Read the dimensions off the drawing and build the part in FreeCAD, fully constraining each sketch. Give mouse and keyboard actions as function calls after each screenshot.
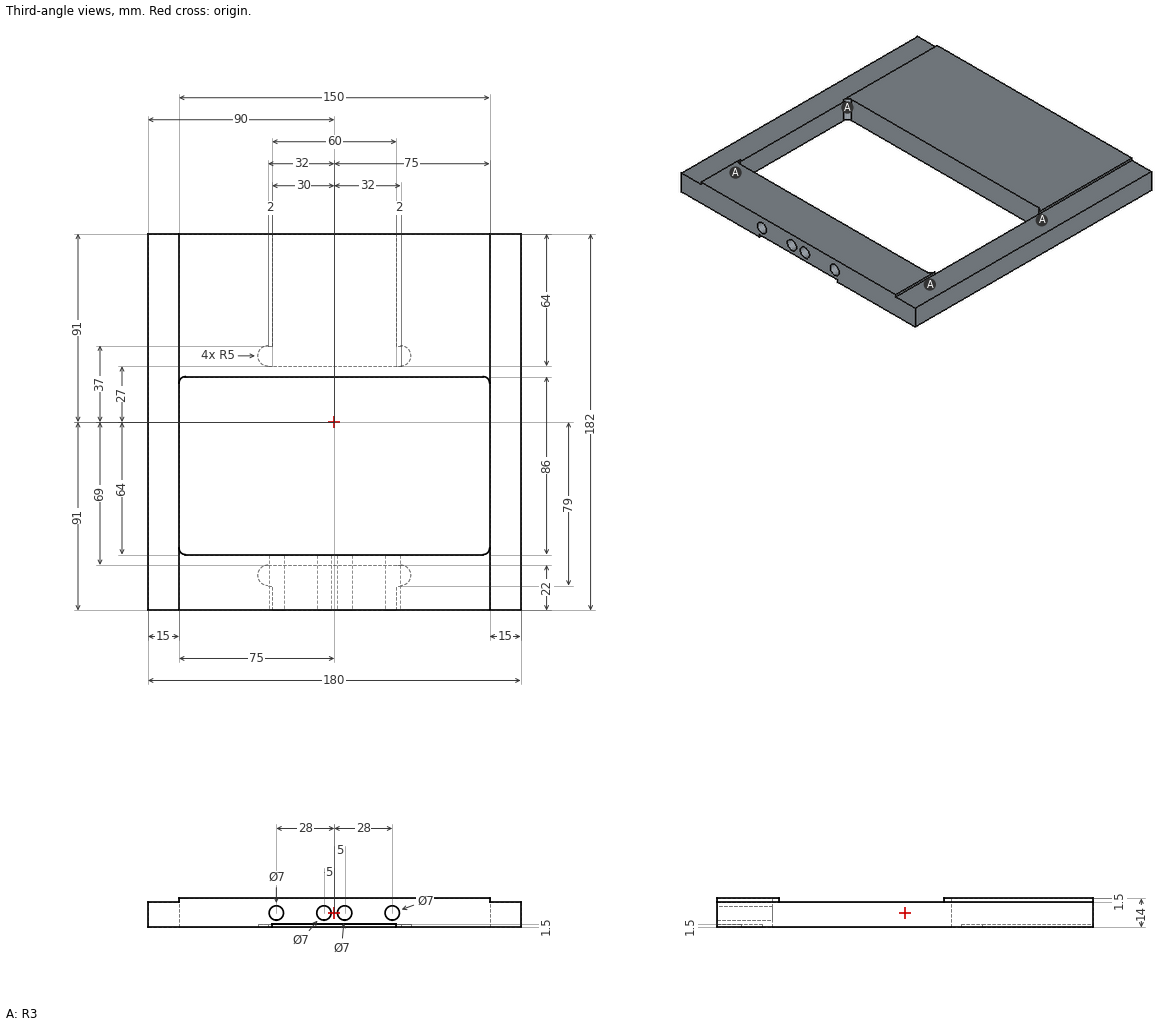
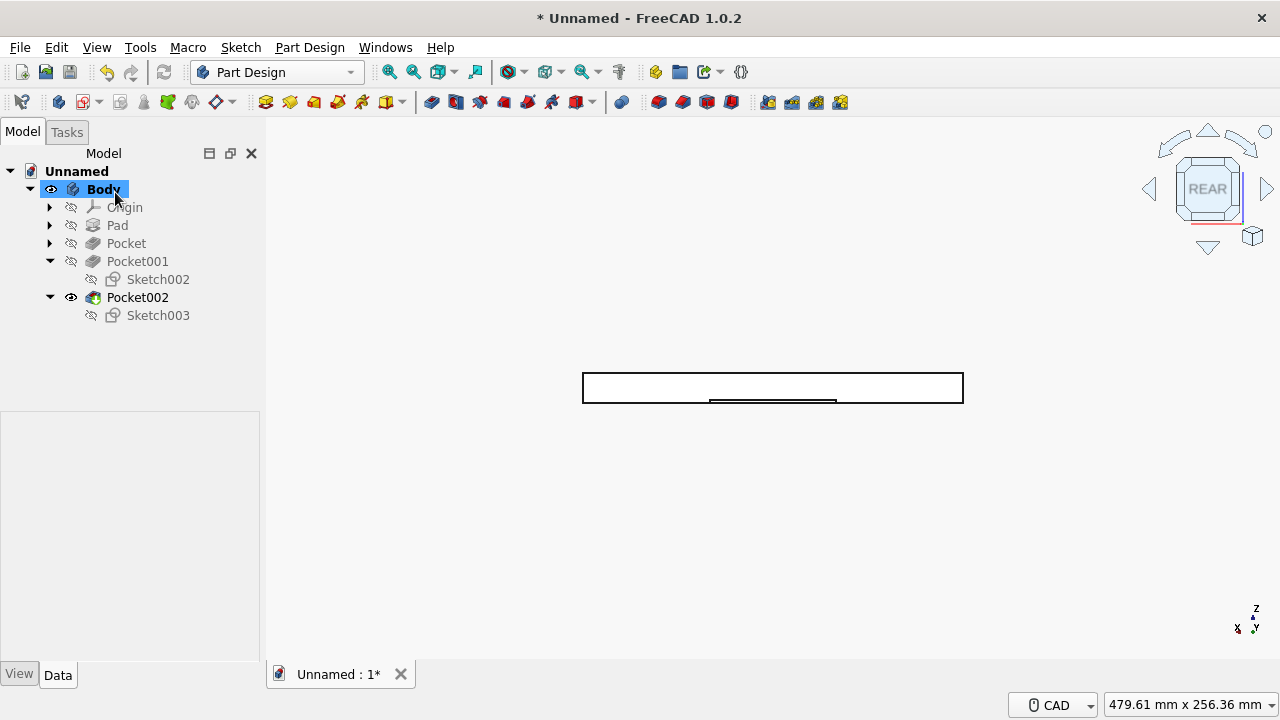
key(6)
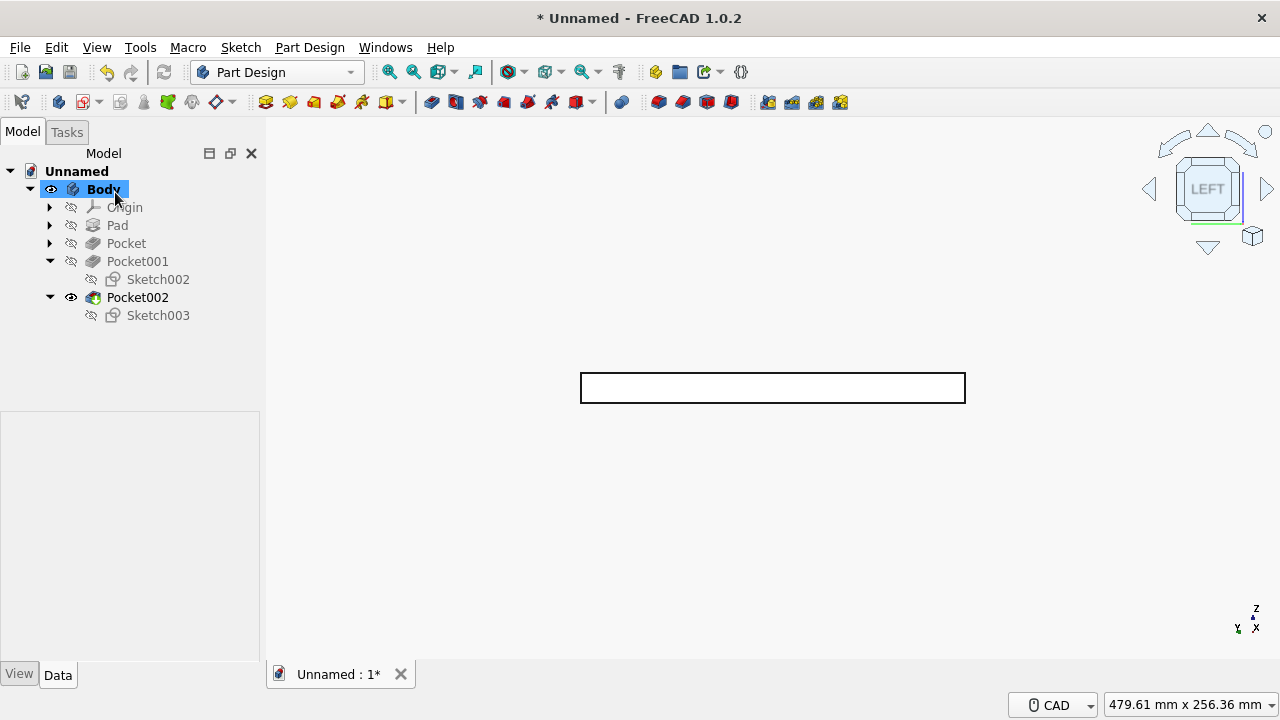
key(v)
key(f)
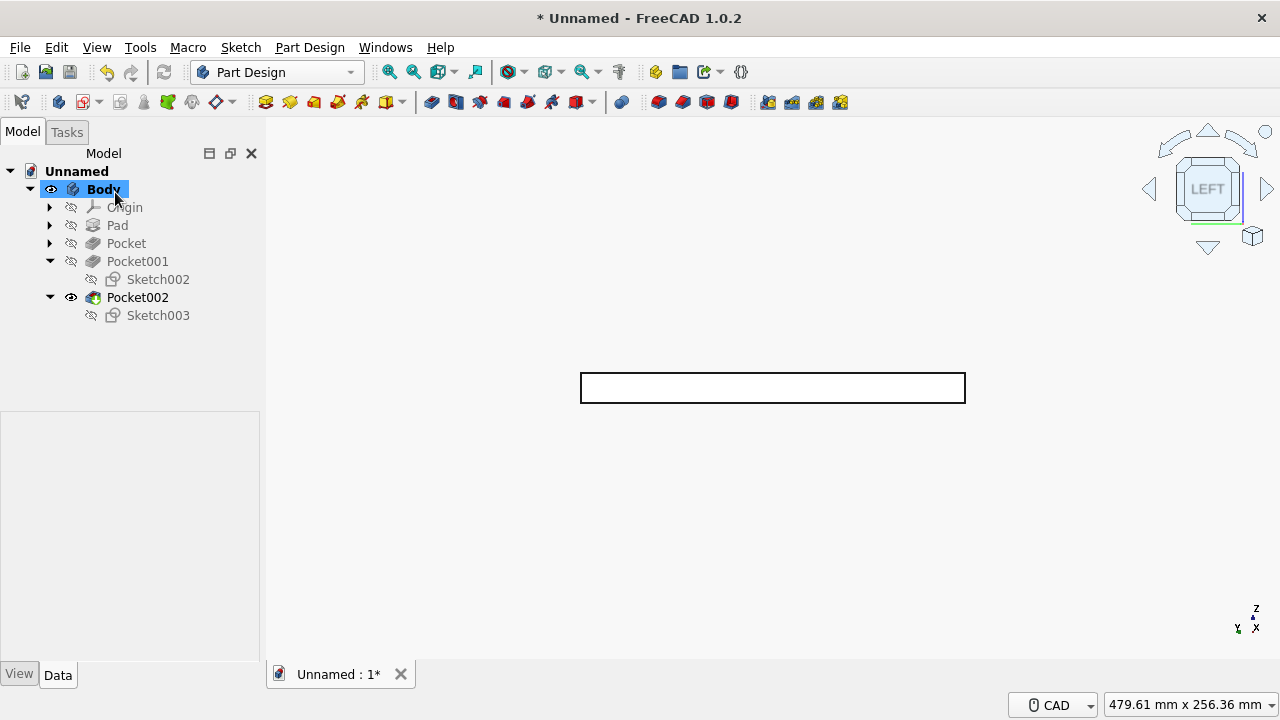
key(v)
key(3)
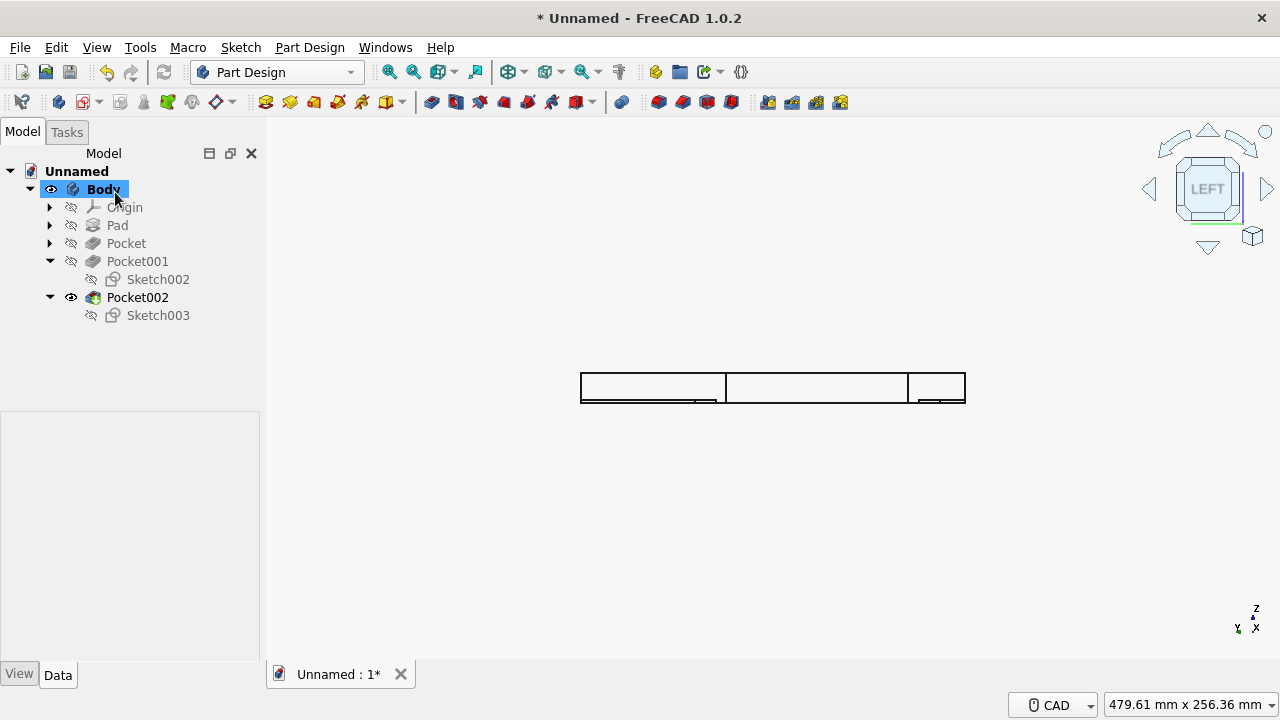
key(0)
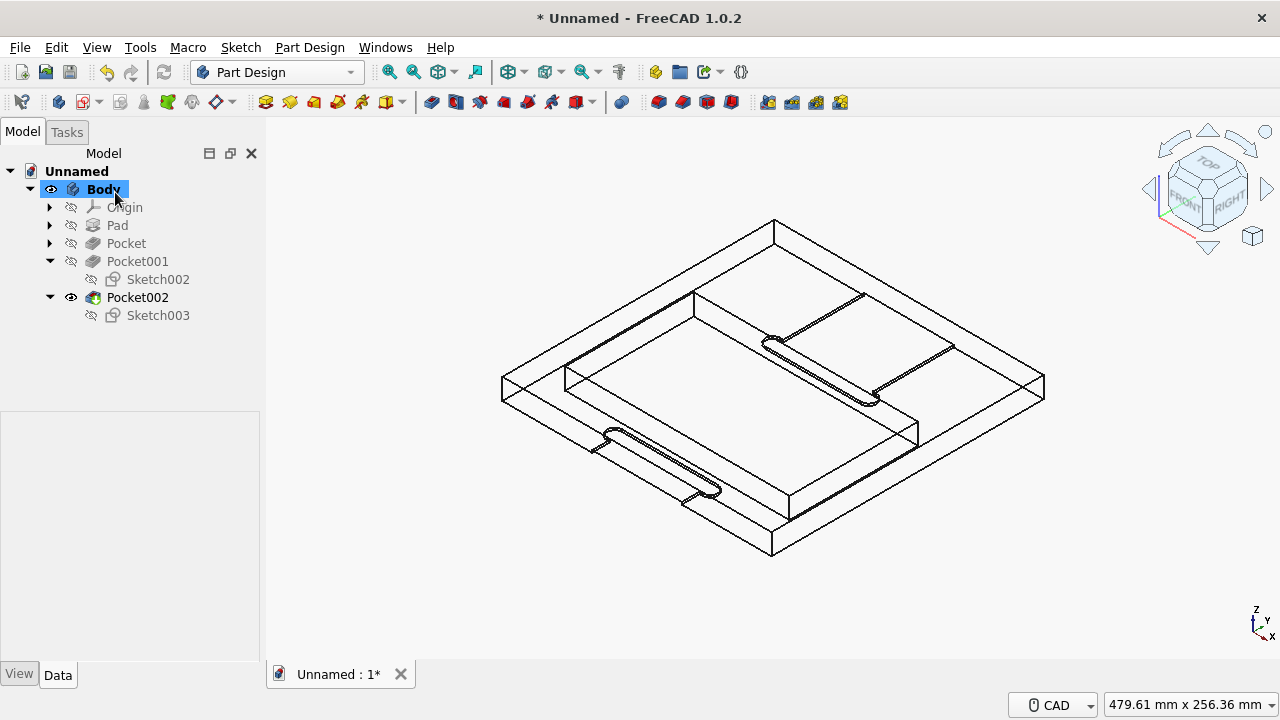
click(694, 303)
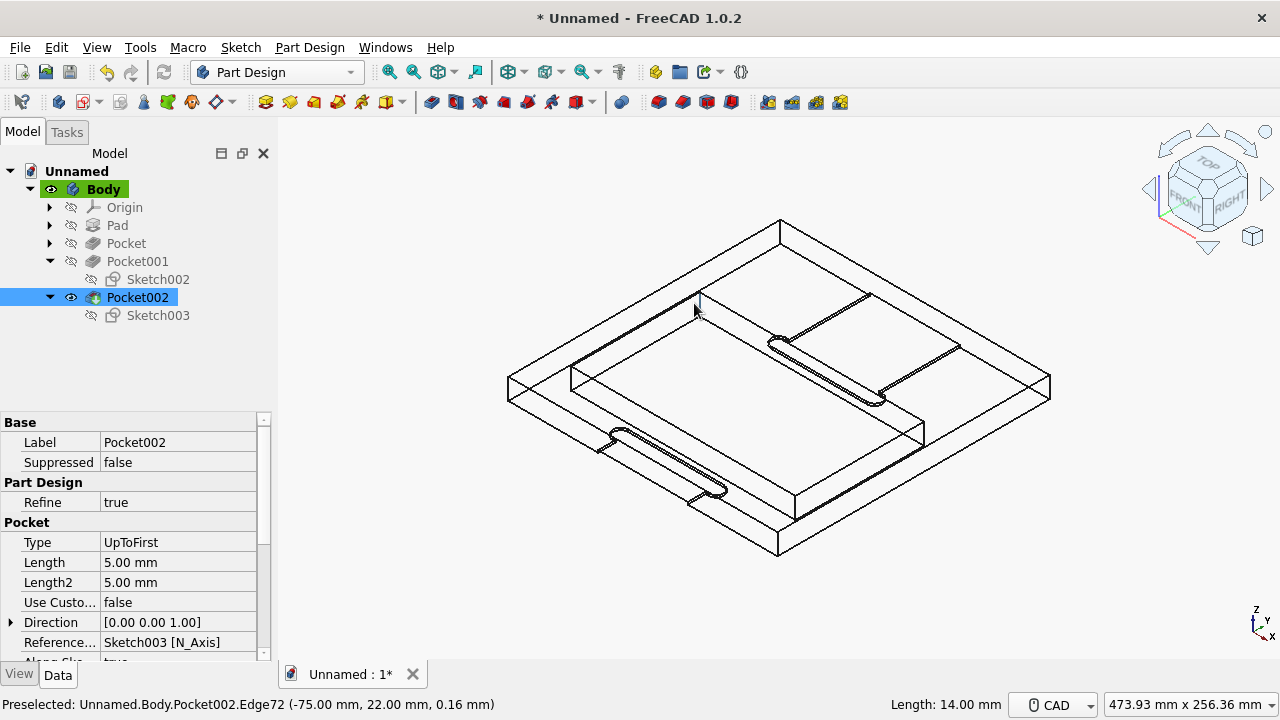
click(571, 378, ctrl)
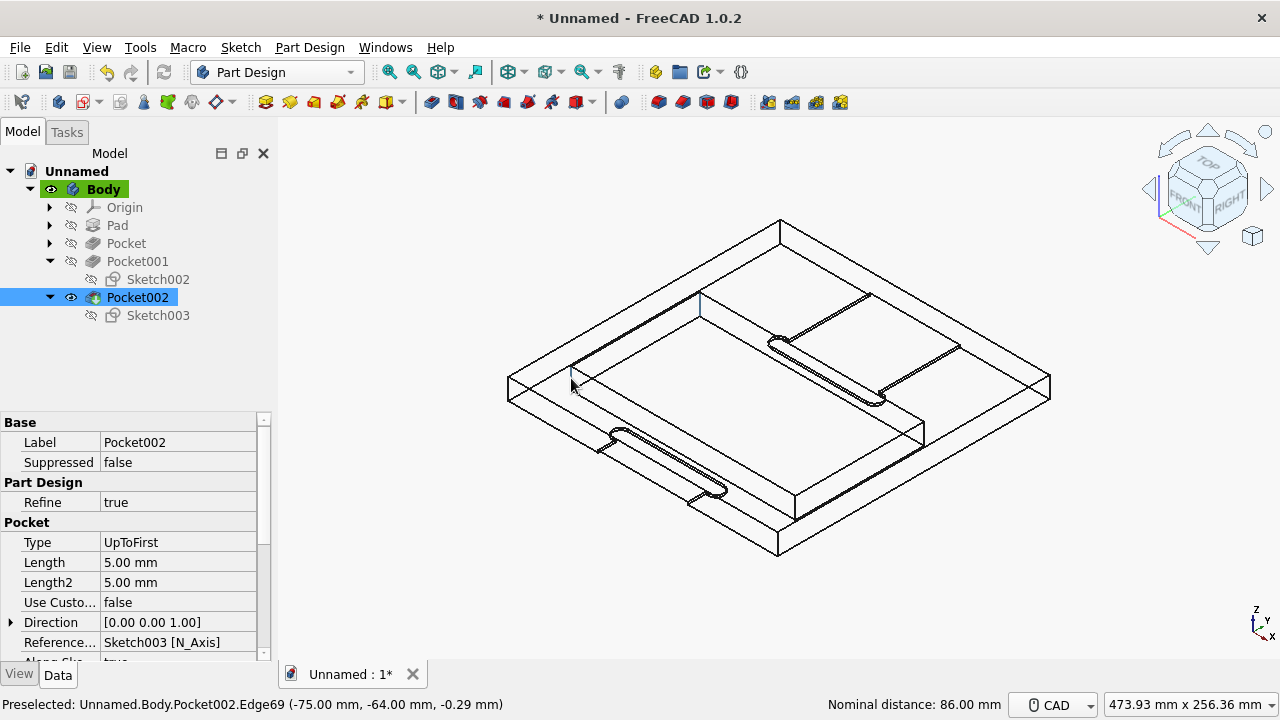
click(795, 507, ctrl)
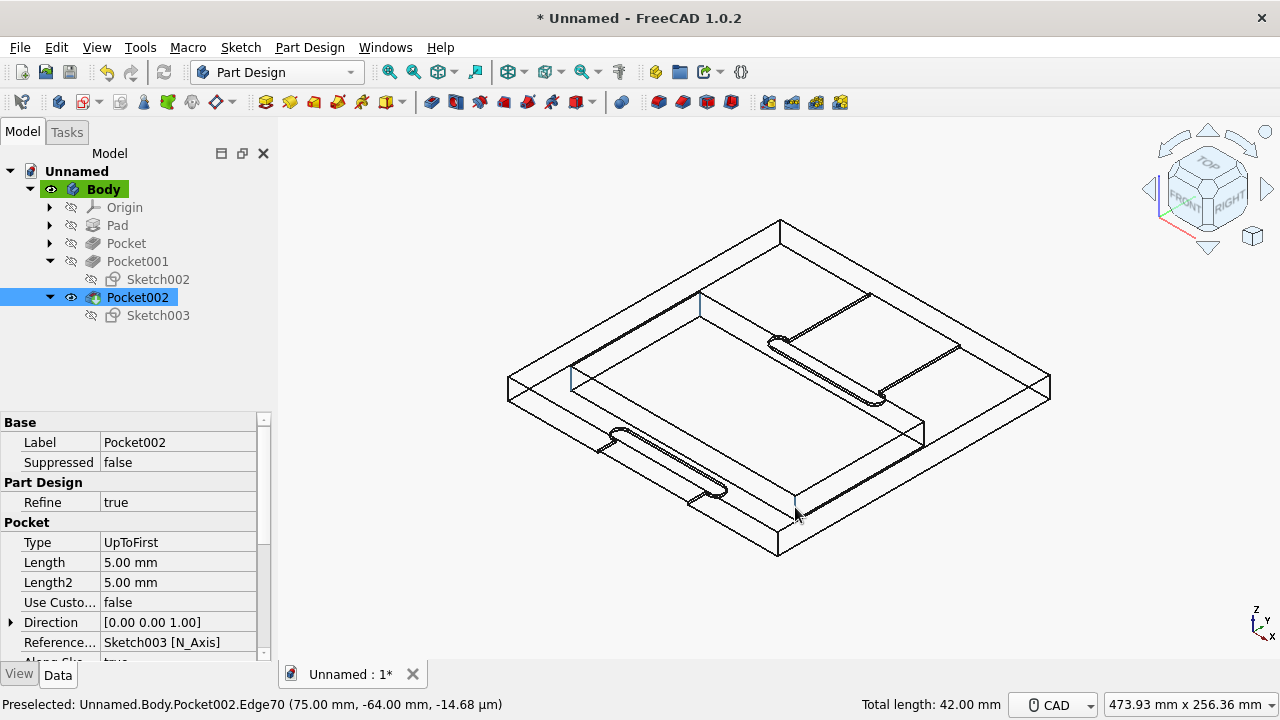
click(924, 433, ctrl)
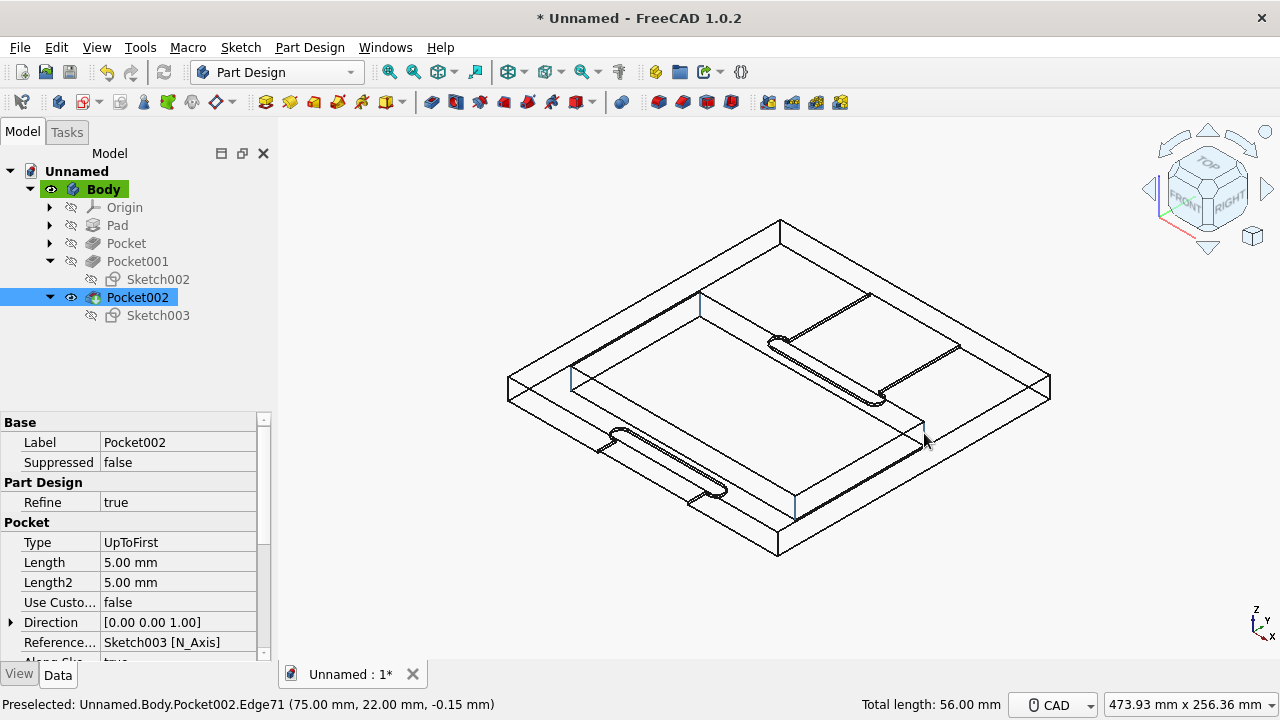
key(v)
key(1)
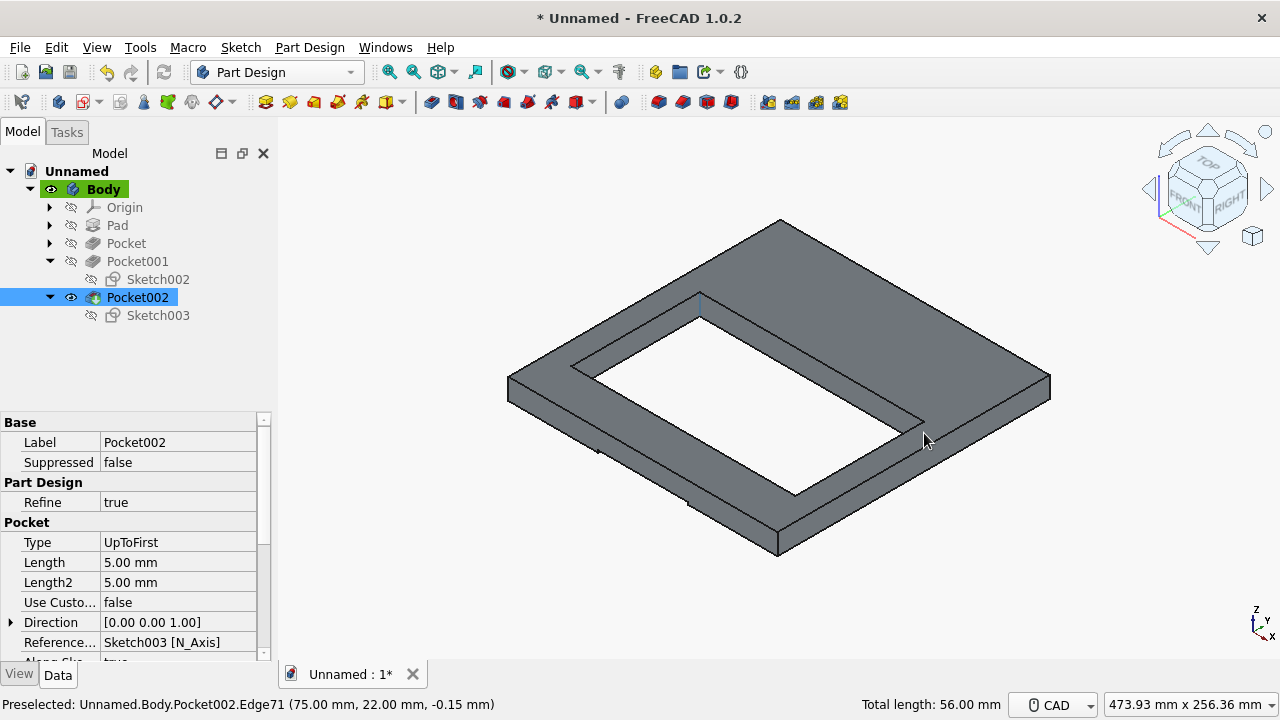
click(660, 102)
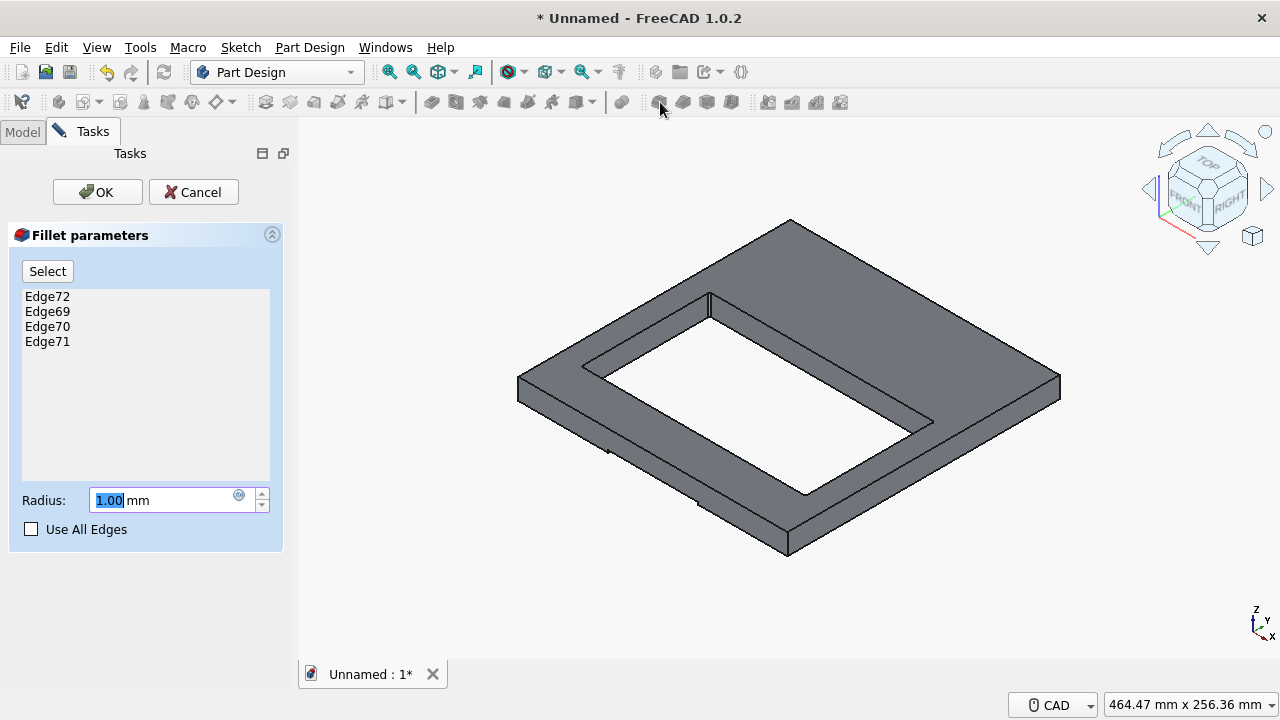
text(3)
key(Tab)